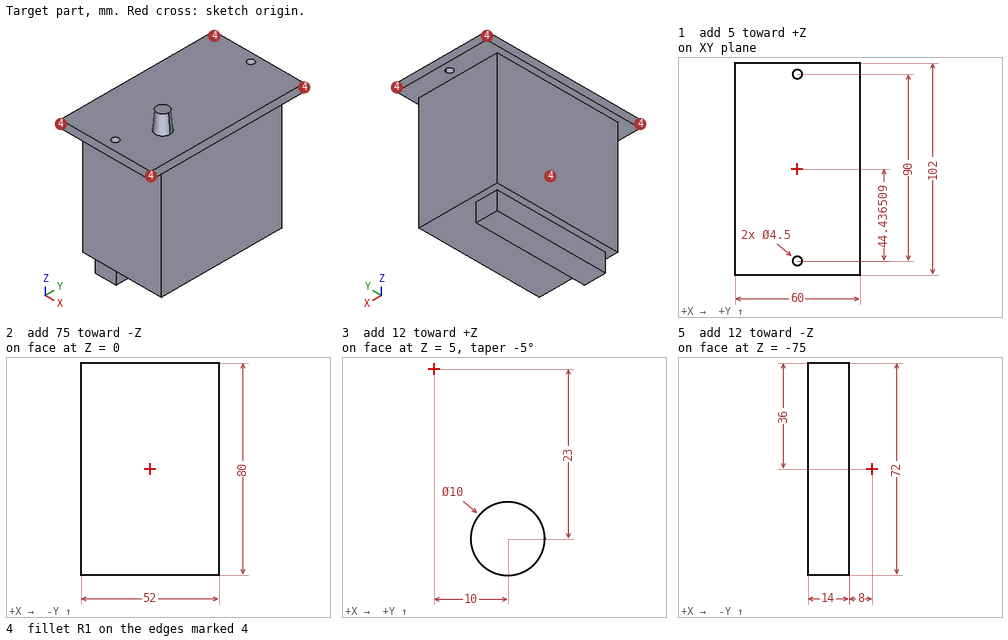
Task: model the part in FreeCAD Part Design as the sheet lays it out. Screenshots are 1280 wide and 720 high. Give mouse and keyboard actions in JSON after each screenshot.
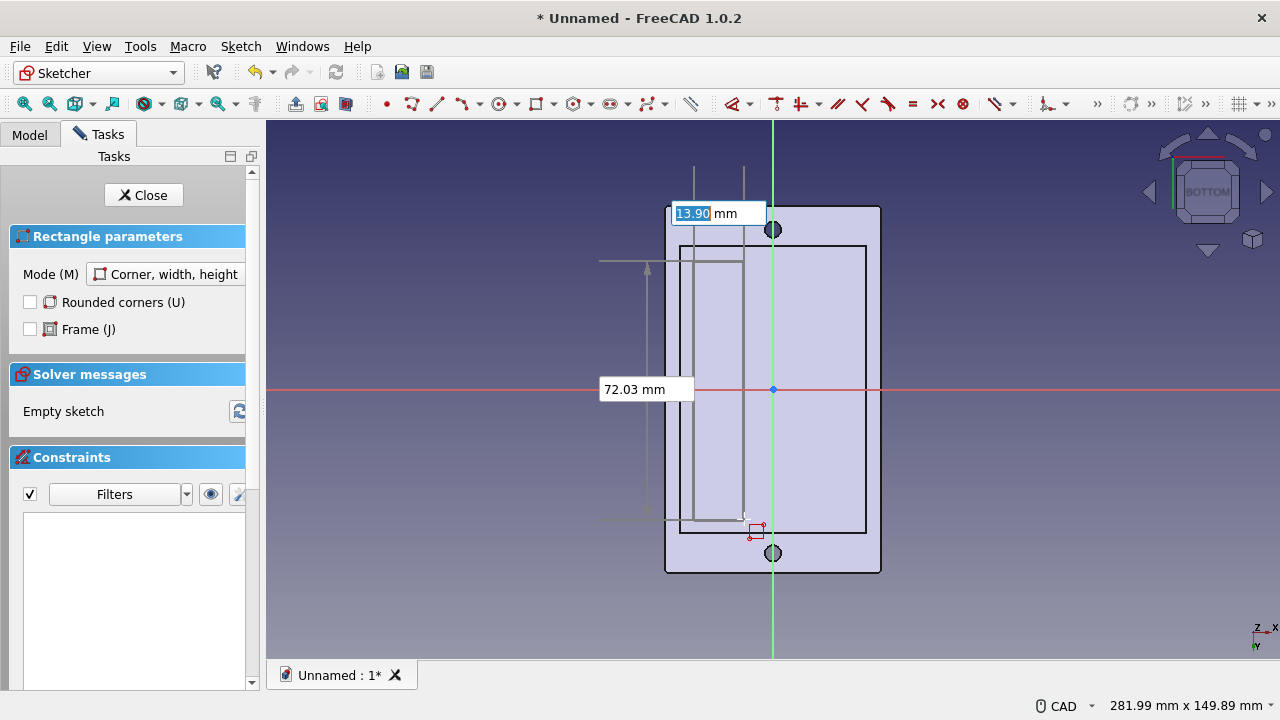
{"action": "type", "text": "14"}
{"action": "key", "text": "Tab"}
{"action": "type", "text": "72"}
{"action": "key", "text": "Return"}
{"action": "key", "text": "Escape"}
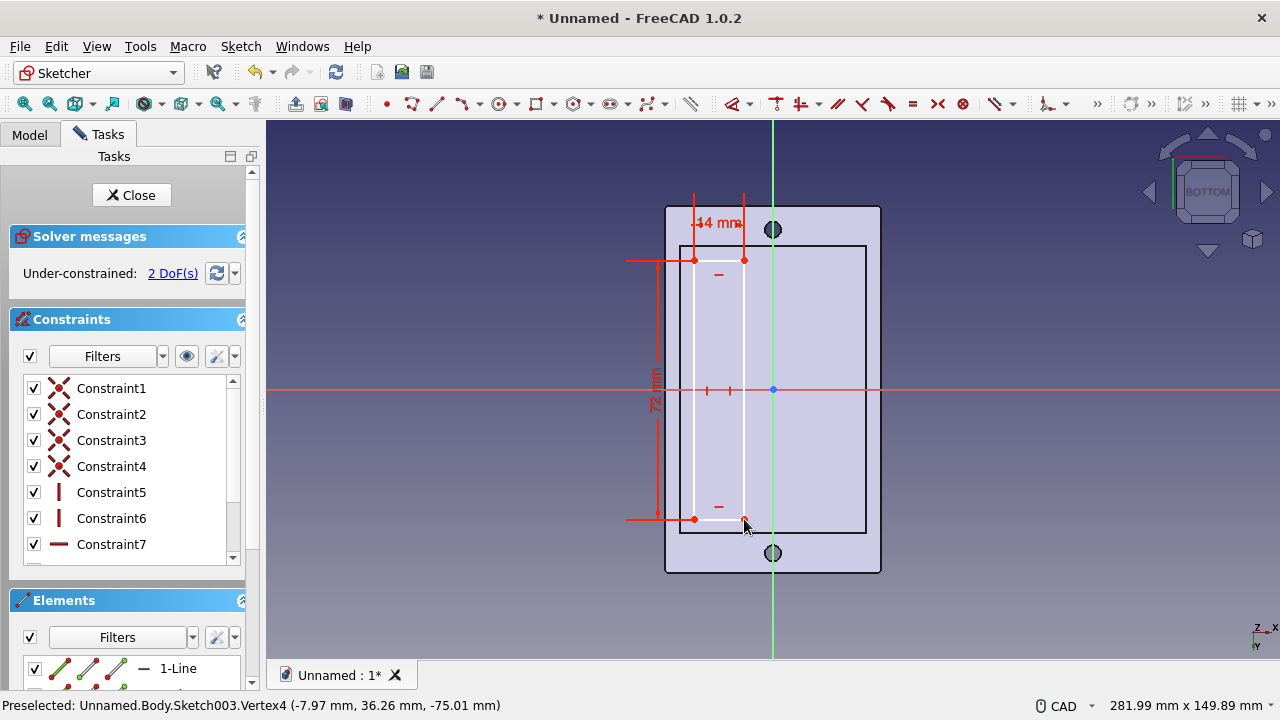
{"action": "left_click", "coordinate": [732, 104]}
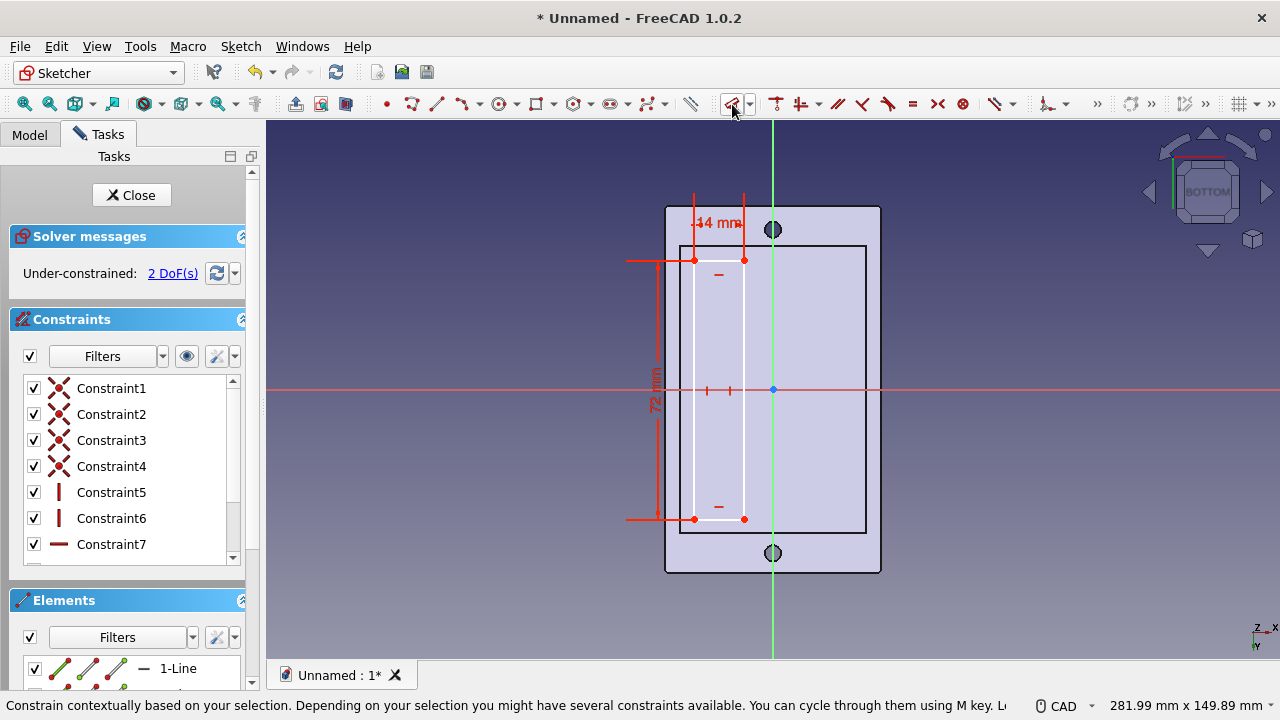
{"action": "scroll", "coordinate": [744, 520], "scroll_direction": "up", "scroll_amount": 2}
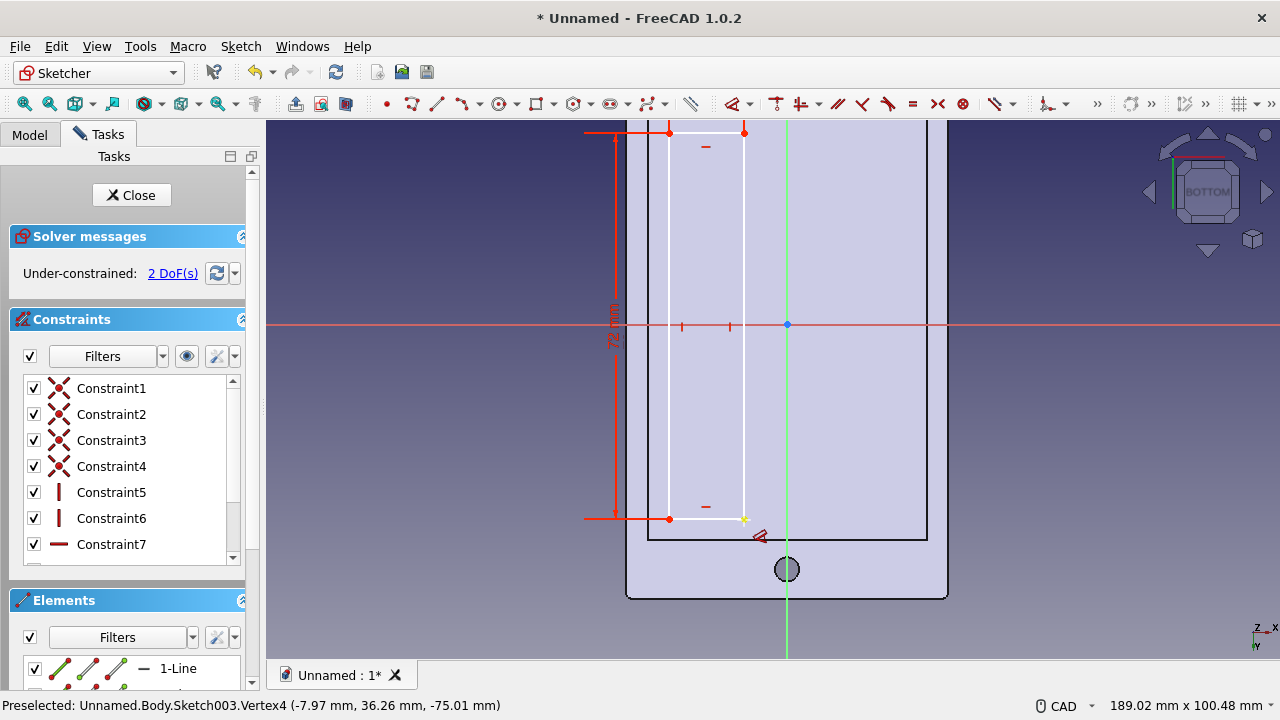
{"action": "left_click", "coordinate": [744, 519]}
{"action": "left_click", "coordinate": [766, 553]}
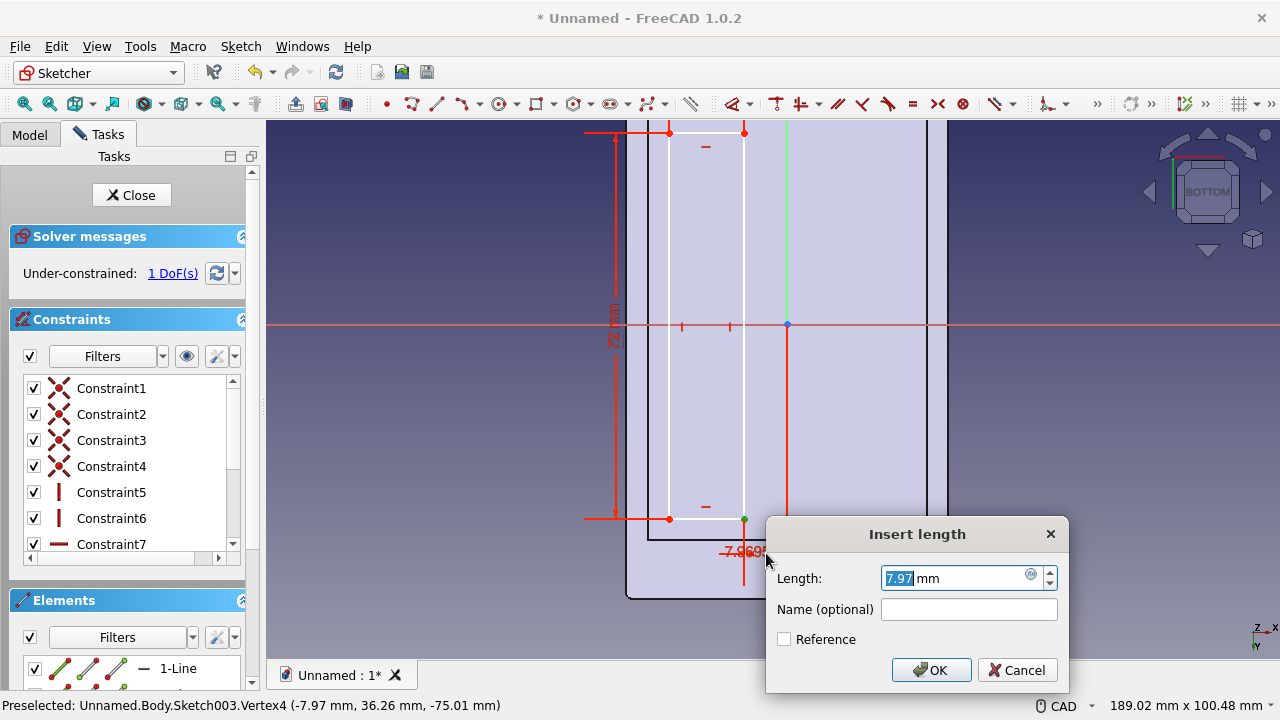
{"action": "type", "text": "8"}
{"action": "key", "text": "Return"}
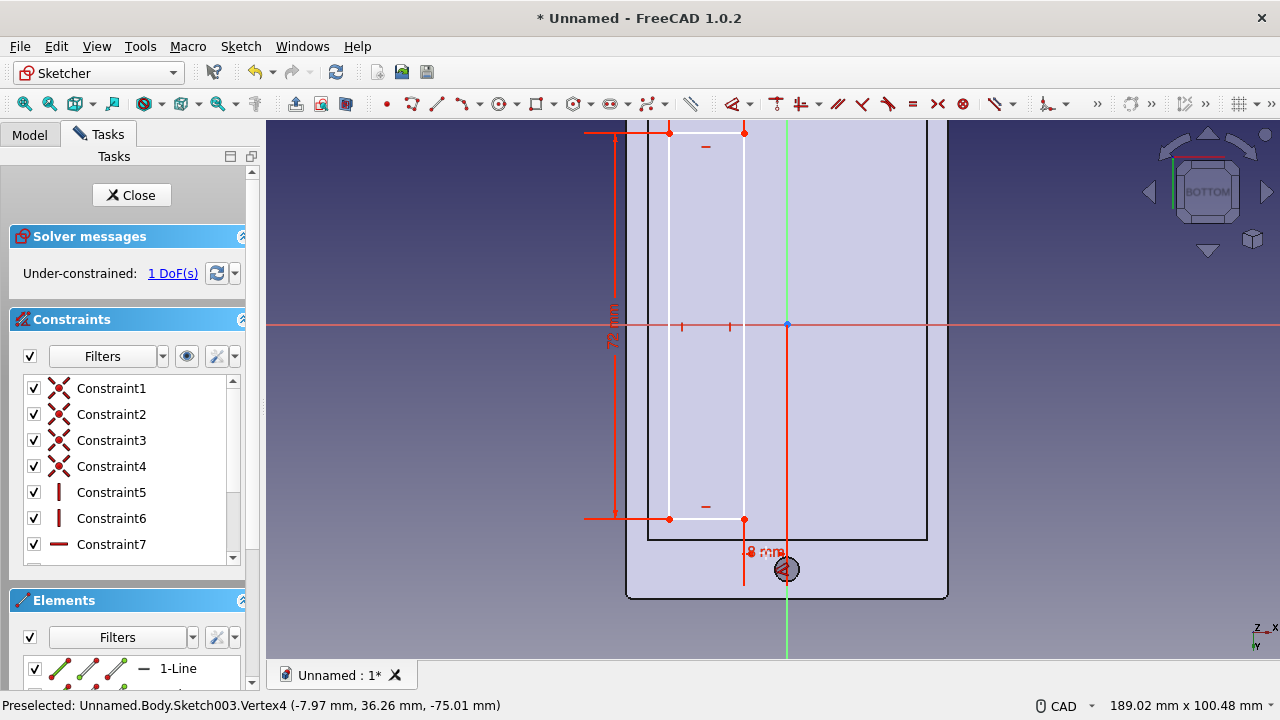
{"action": "scroll", "coordinate": [598, 631], "scroll_direction": "down", "scroll_amount": 1}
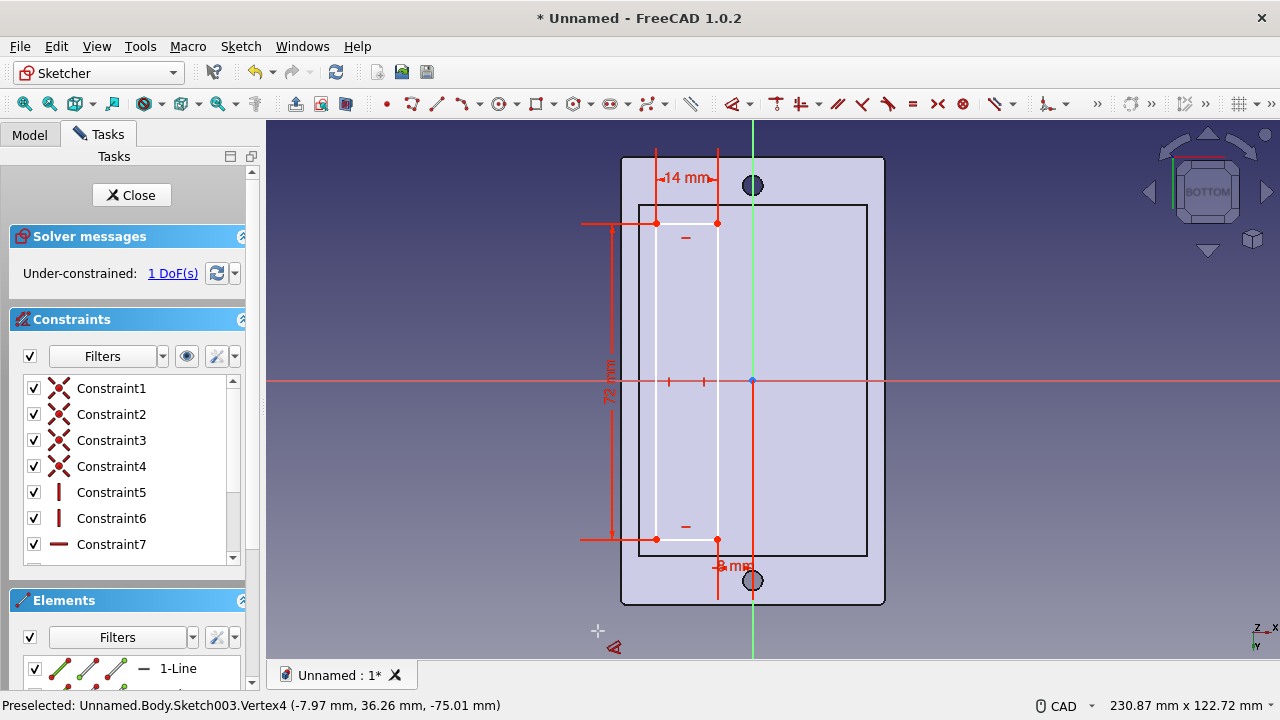
{"action": "left_click", "coordinate": [656, 224]}
{"action": "left_click", "coordinate": [787, 302]}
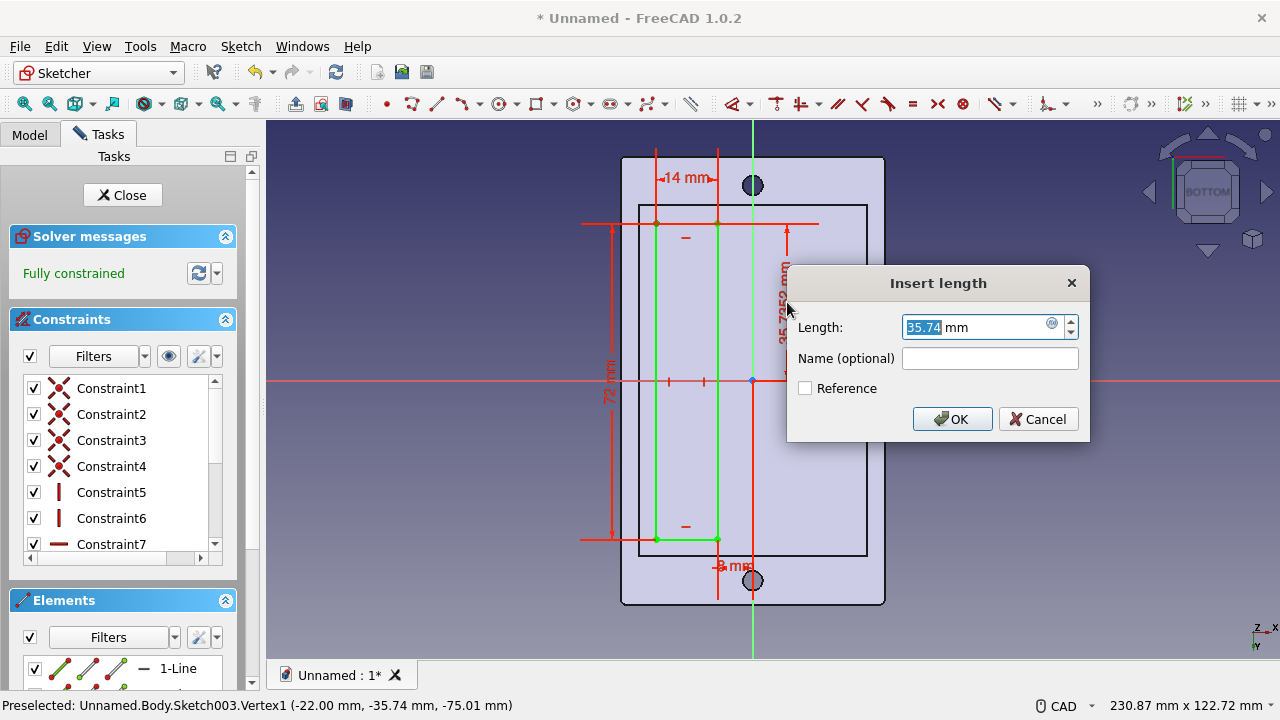
{"action": "type", "text": "36"}
{"action": "key", "text": "Return"}
{"action": "key", "text": "Escape"}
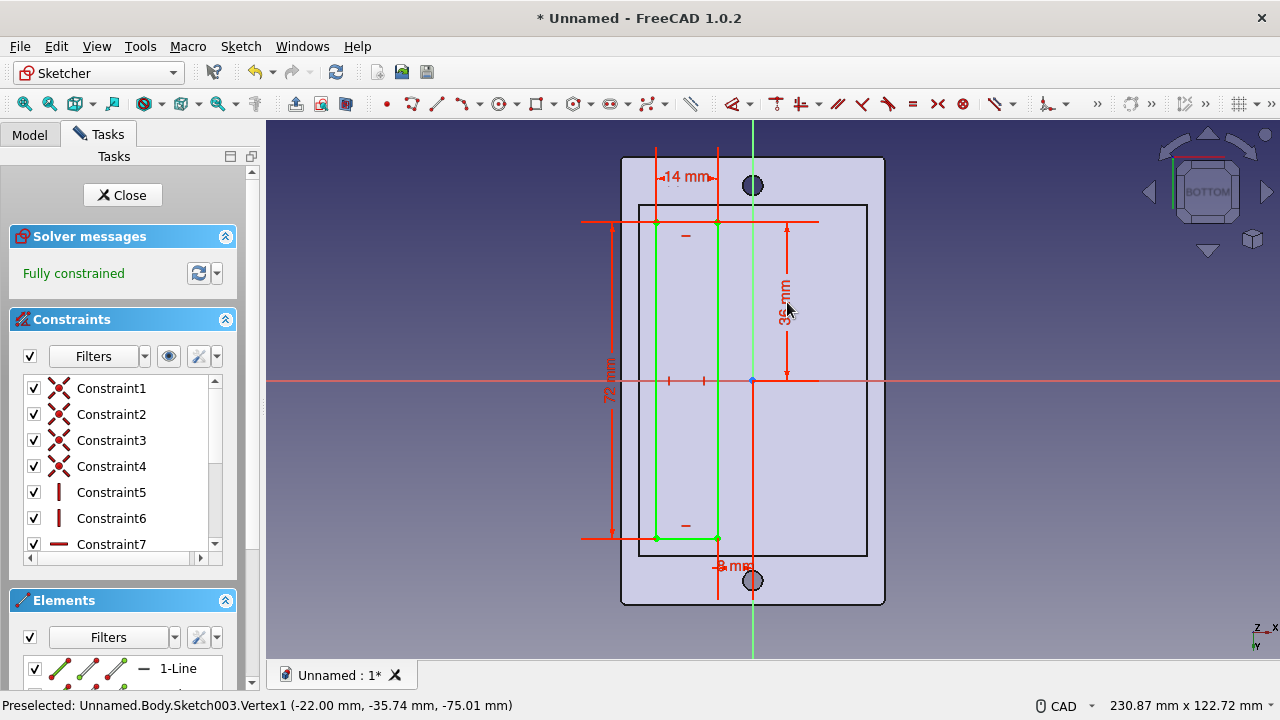
{"action": "left_click", "coordinate": [123, 195]}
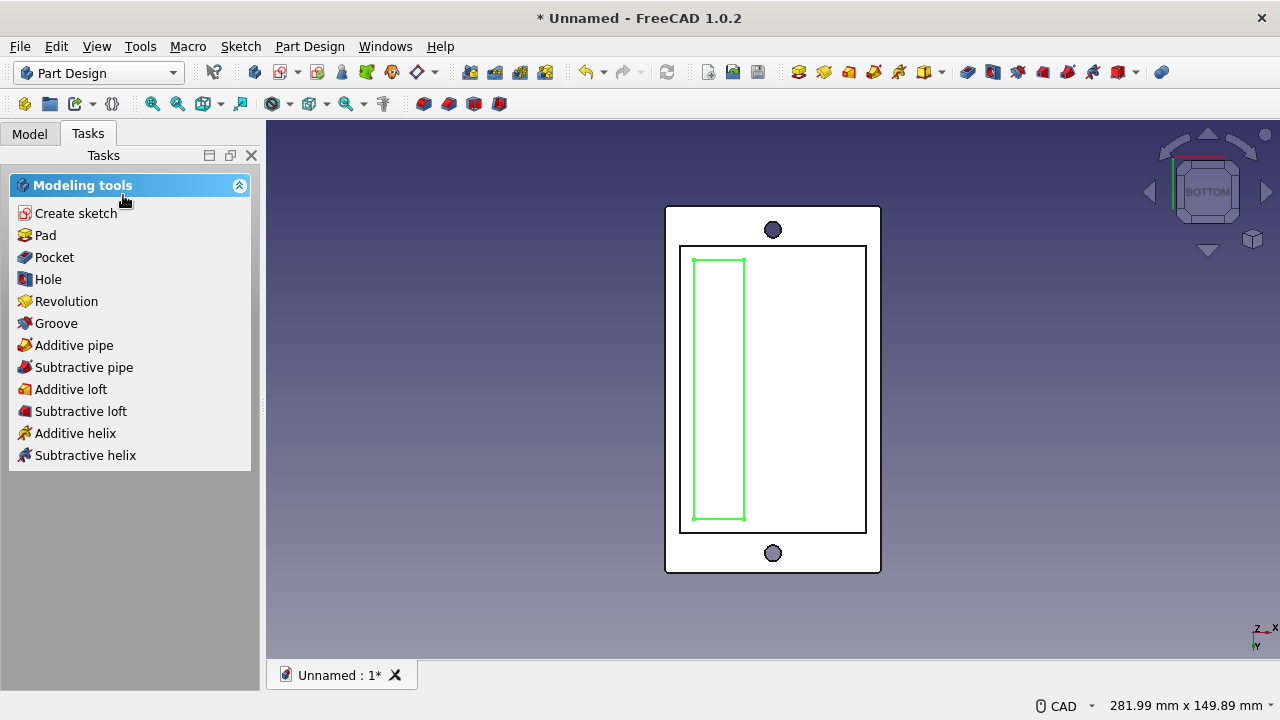
{"action": "left_click", "coordinate": [799, 72]}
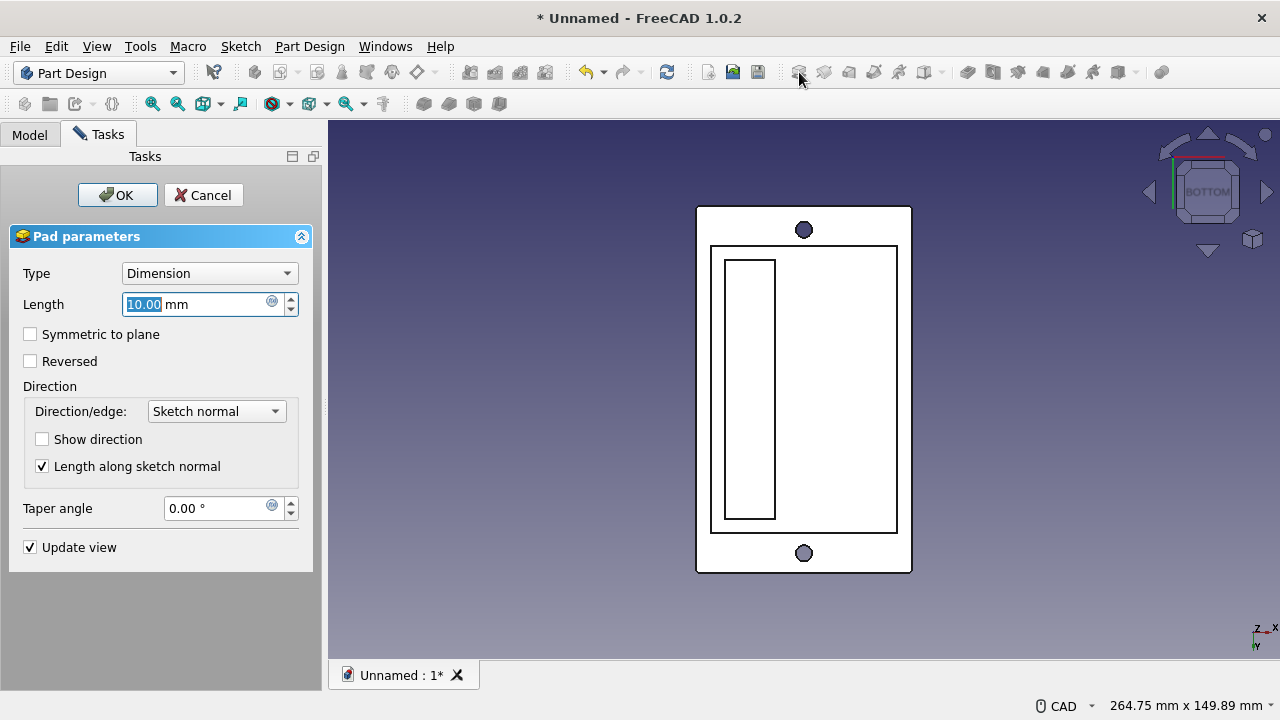
{"action": "type", "text": "12"}
{"action": "key", "text": "Tab"}